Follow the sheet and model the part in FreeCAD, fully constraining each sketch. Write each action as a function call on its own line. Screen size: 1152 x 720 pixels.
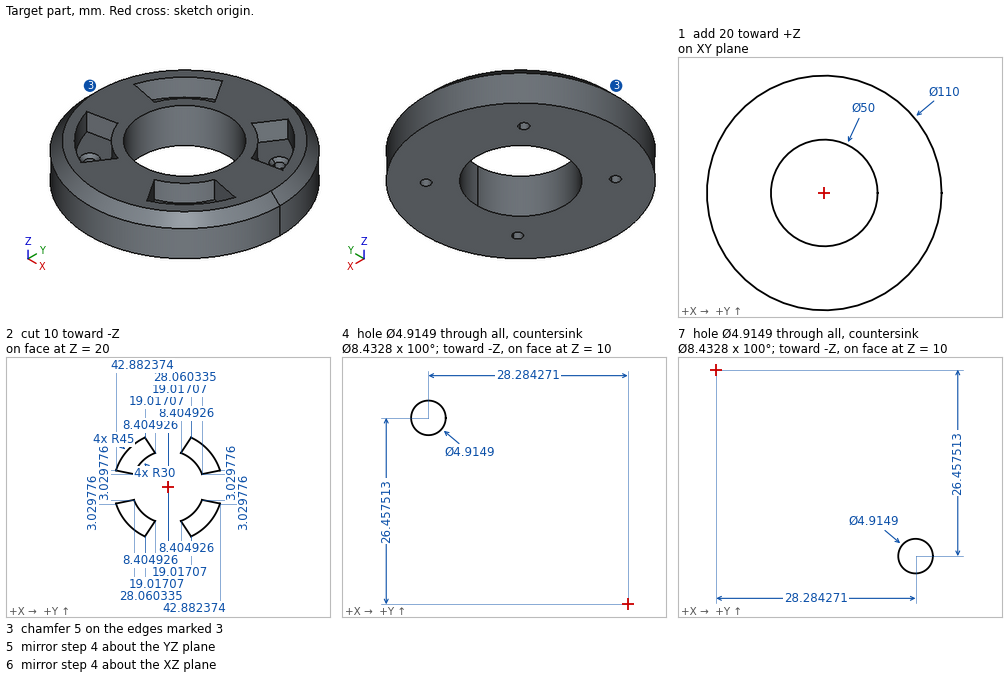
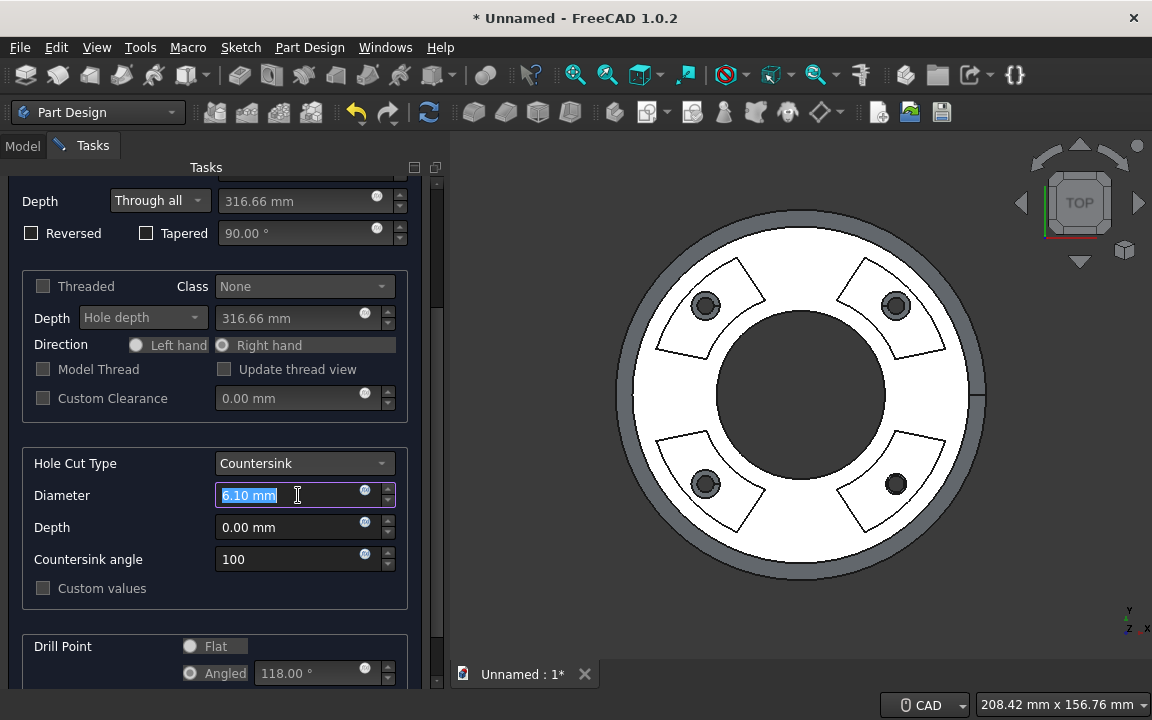
text(8.4328)
key(Tab)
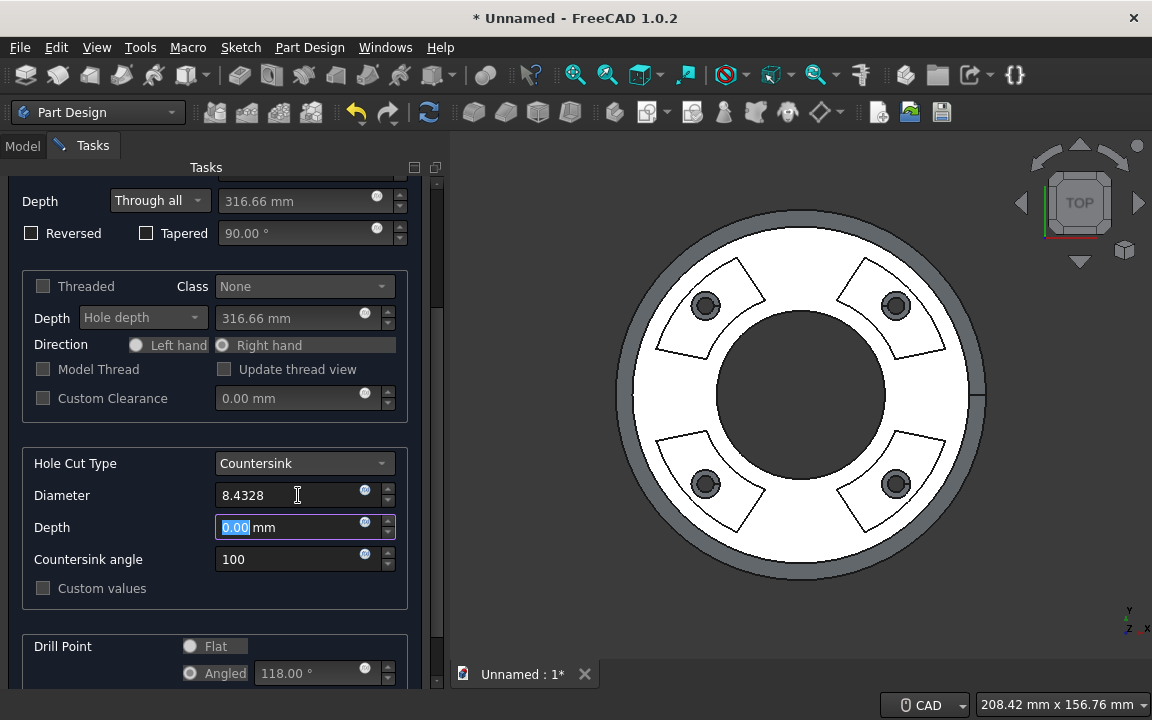
scroll(437, 432, up, 4)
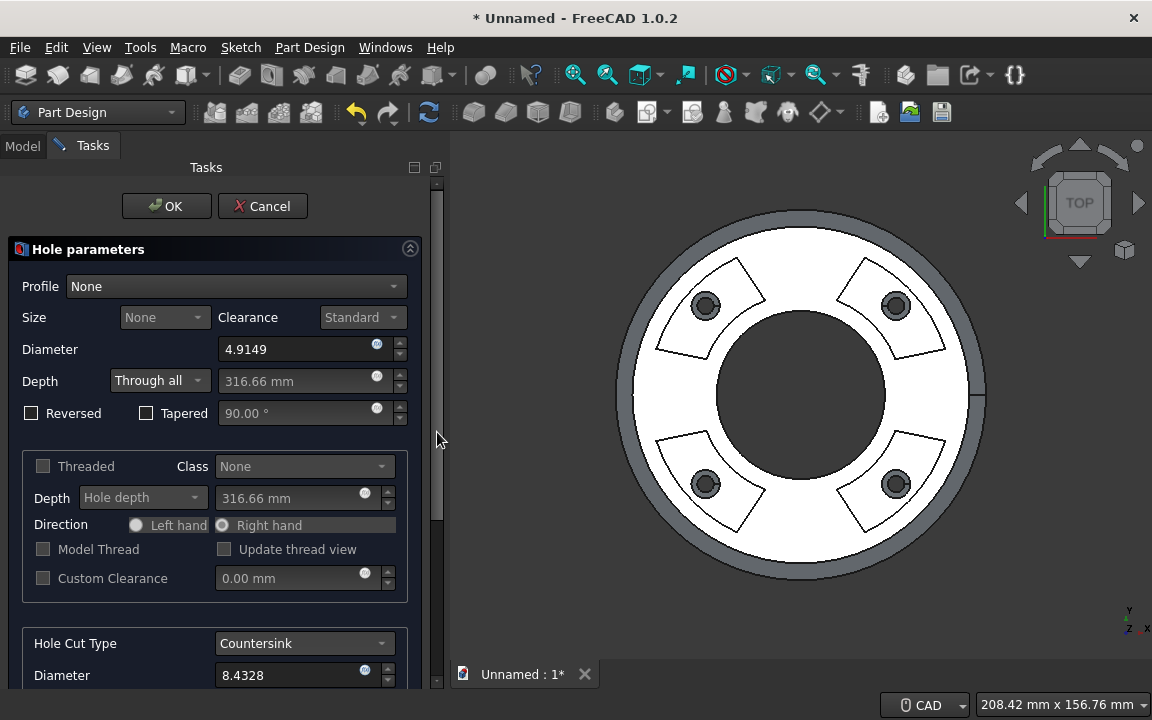
click(167, 206)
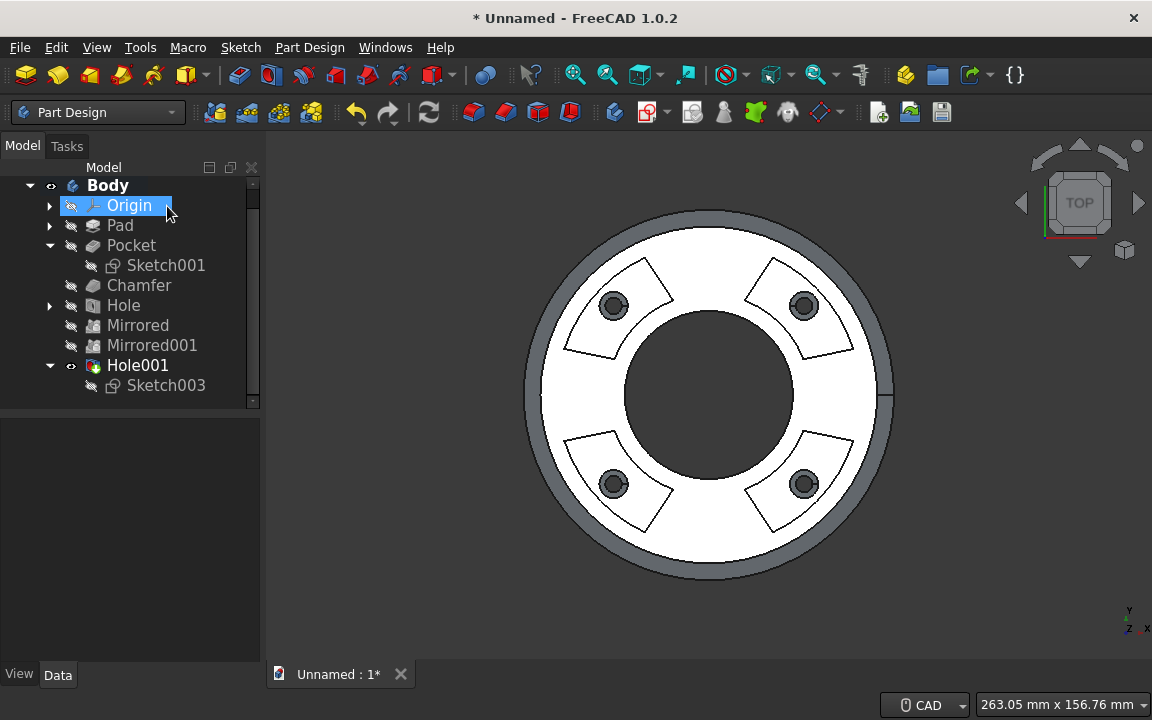
key(0)